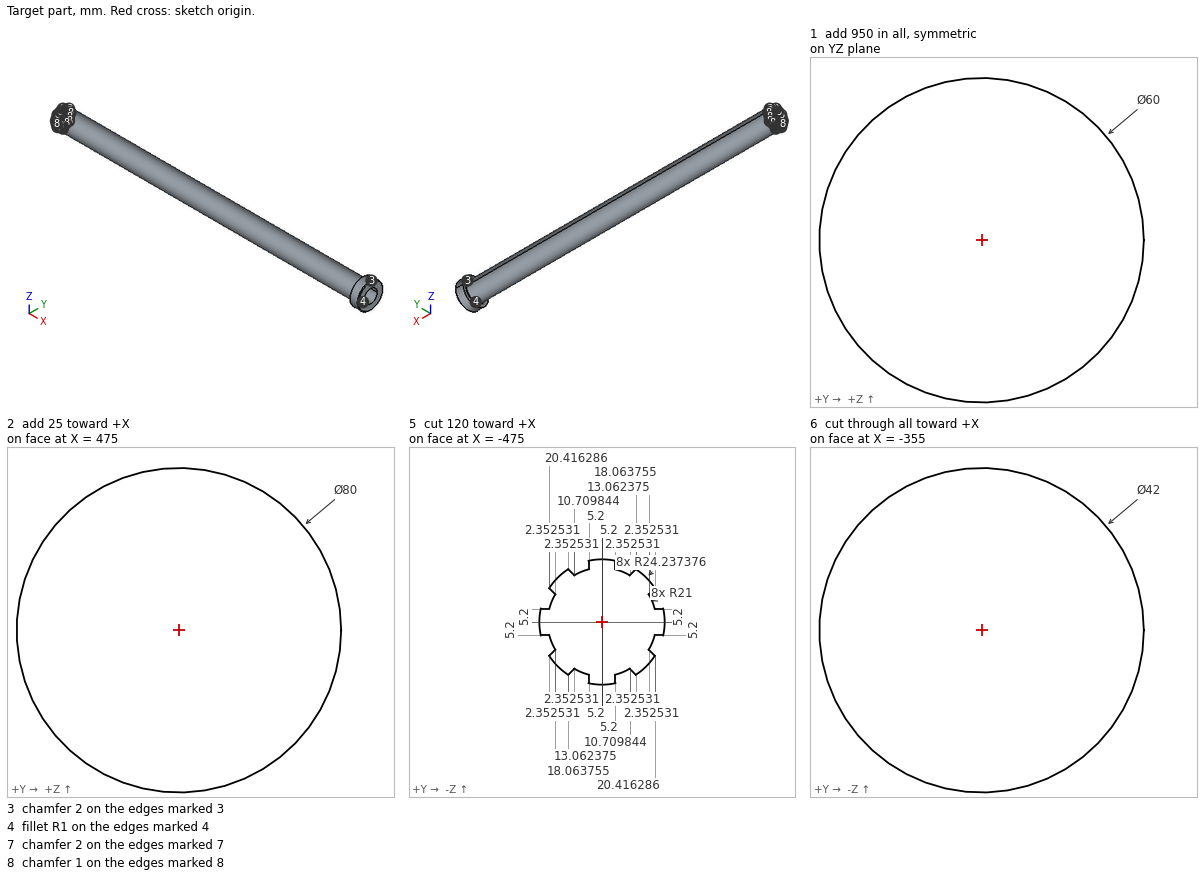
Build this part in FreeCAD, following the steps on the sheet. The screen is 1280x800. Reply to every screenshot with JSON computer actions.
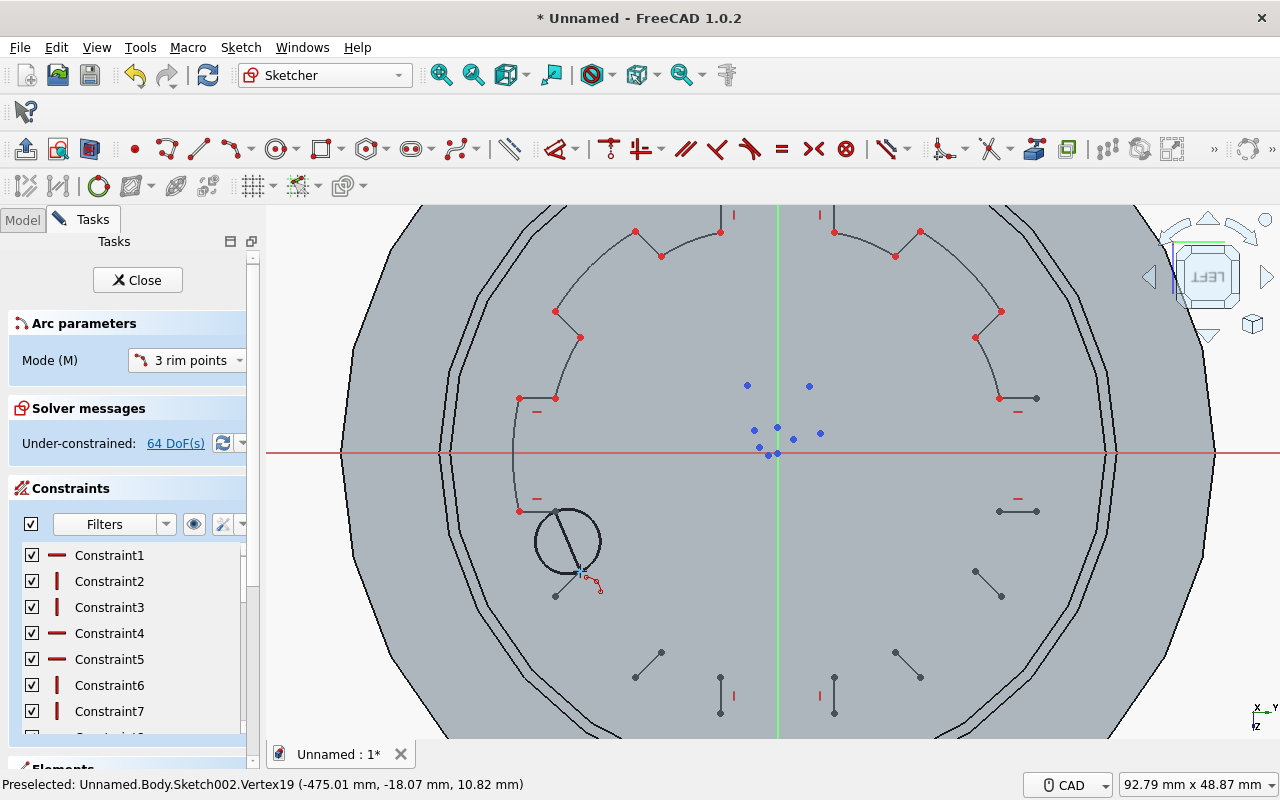
{"action": "scroll", "coordinate": [566, 541], "scroll_direction": "up", "scroll_amount": 10}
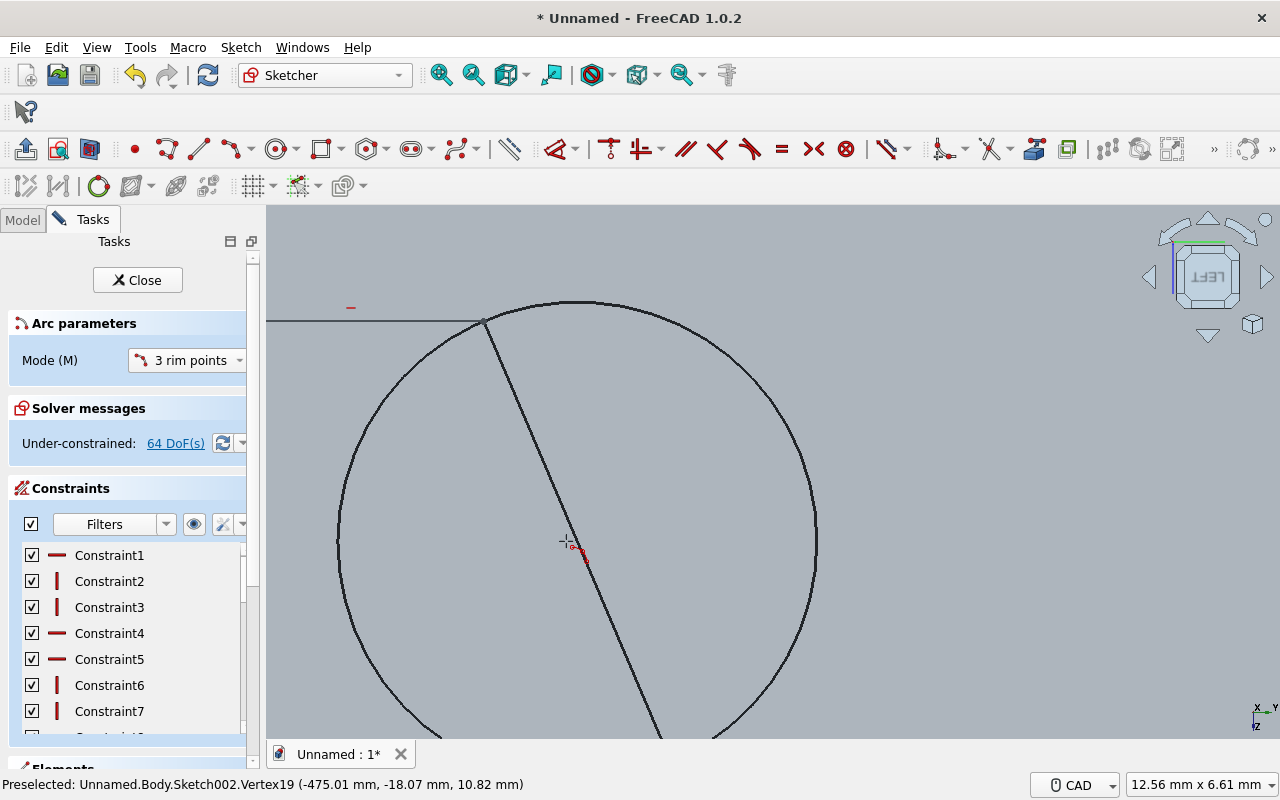
{"action": "left_click", "coordinate": [564, 537]}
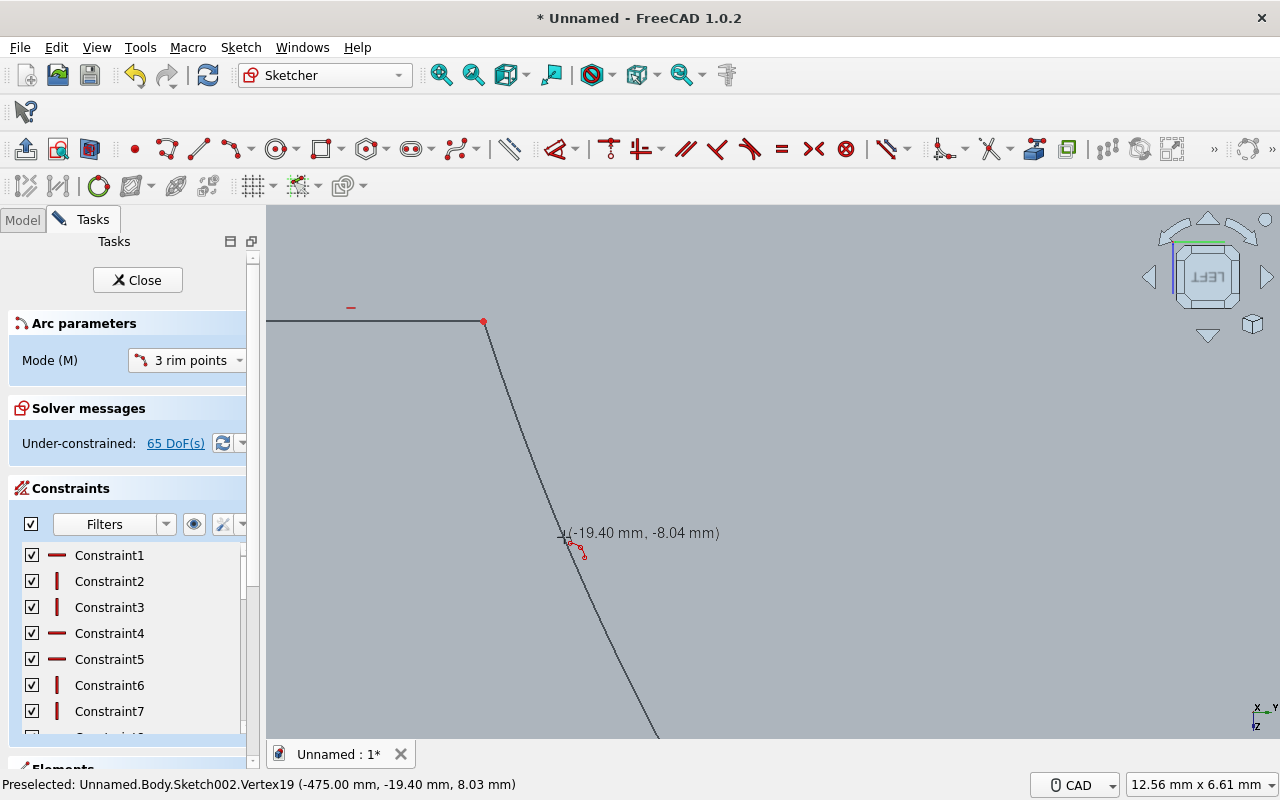
{"action": "scroll", "coordinate": [562, 530], "scroll_direction": "down", "scroll_amount": 12}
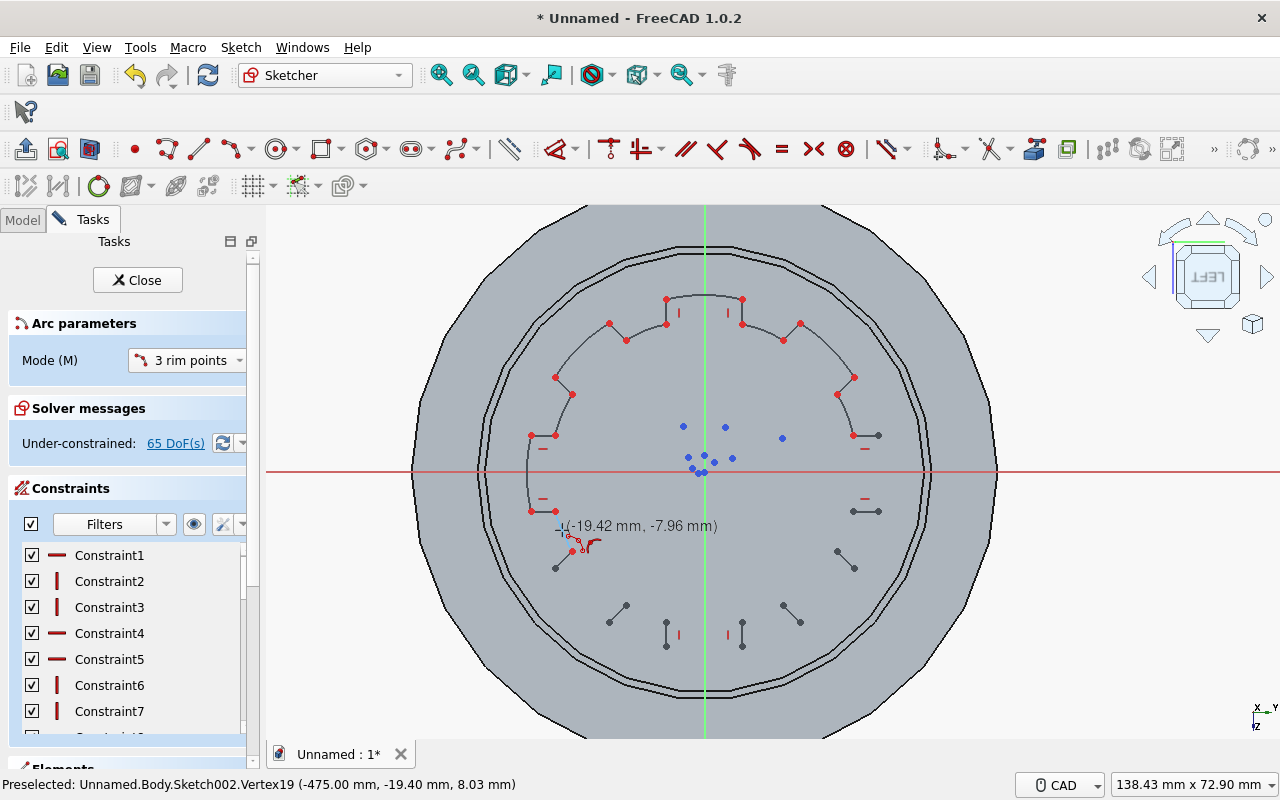
{"action": "scroll", "coordinate": [555, 568], "scroll_direction": "up", "scroll_amount": 2}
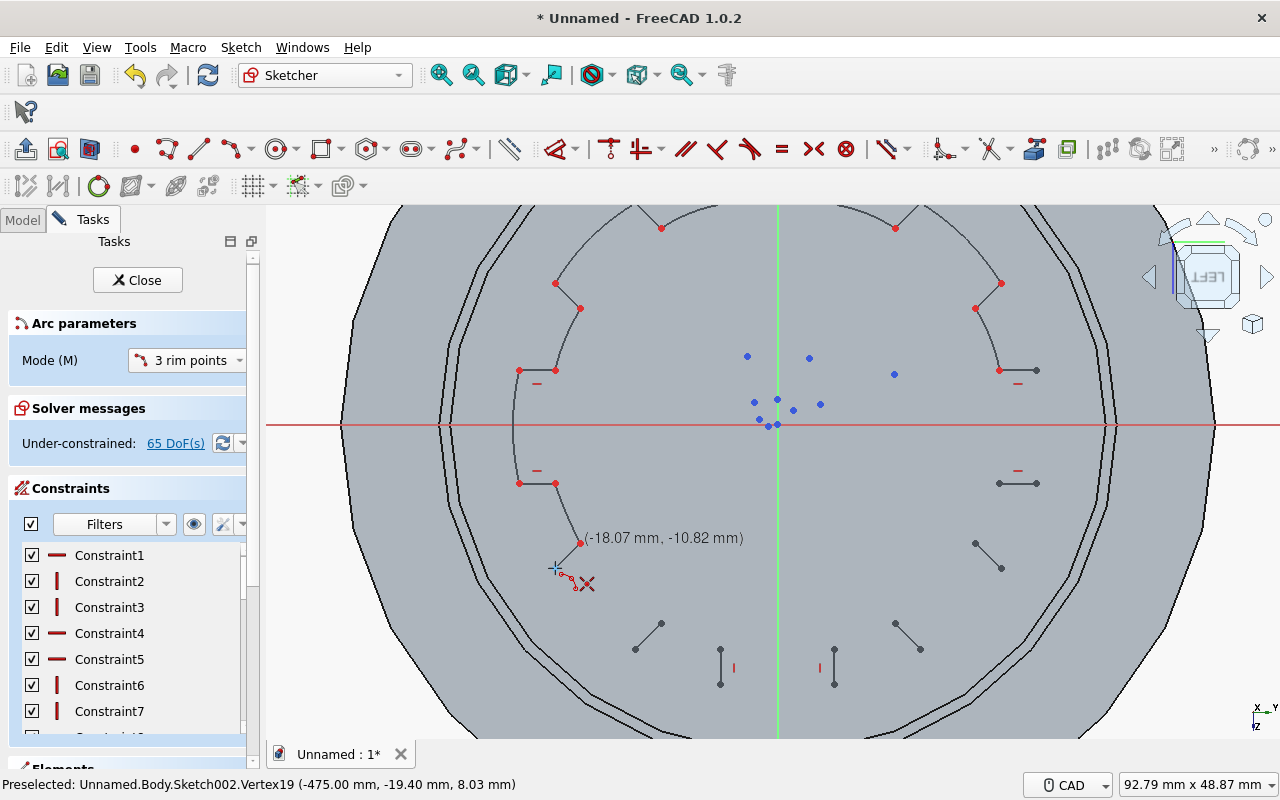
{"action": "left_click", "coordinate": [555, 569]}
{"action": "left_click", "coordinate": [636, 649]}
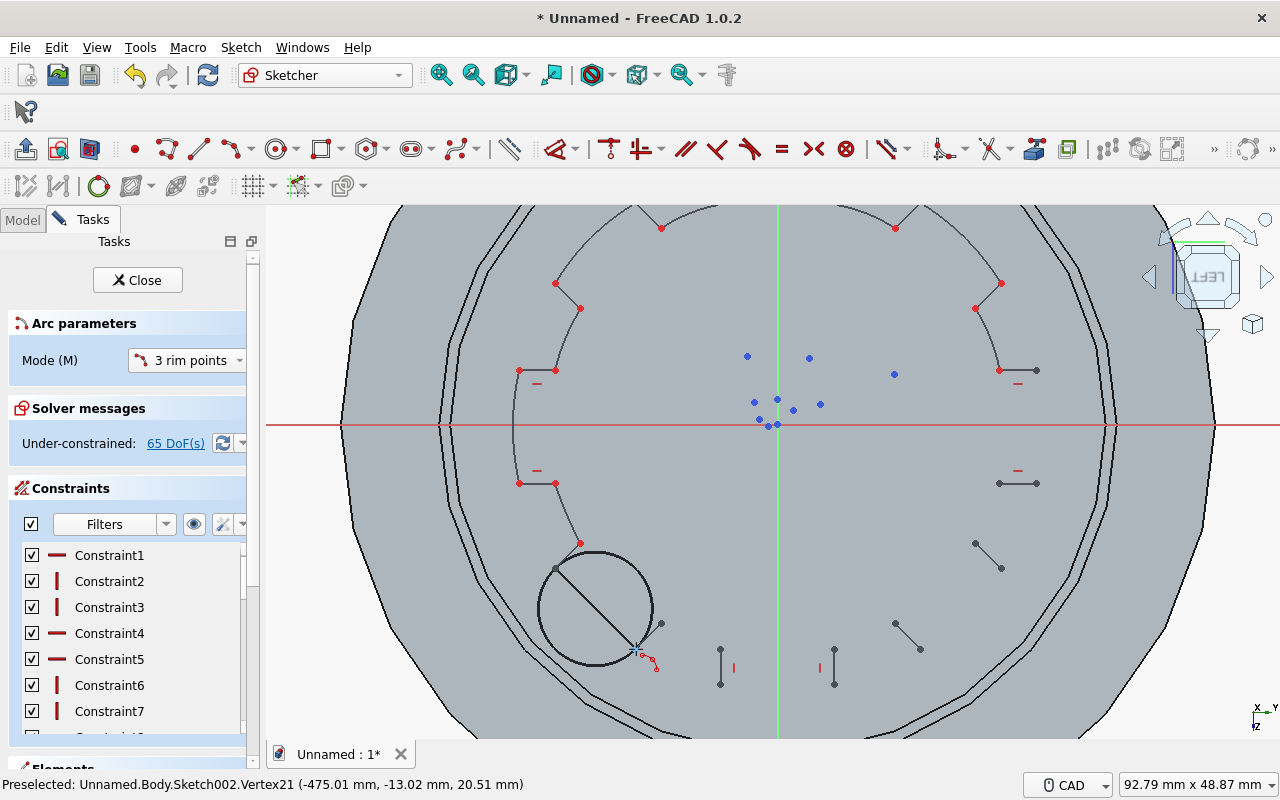
{"action": "scroll", "coordinate": [591, 612], "scroll_direction": "up", "scroll_amount": 5}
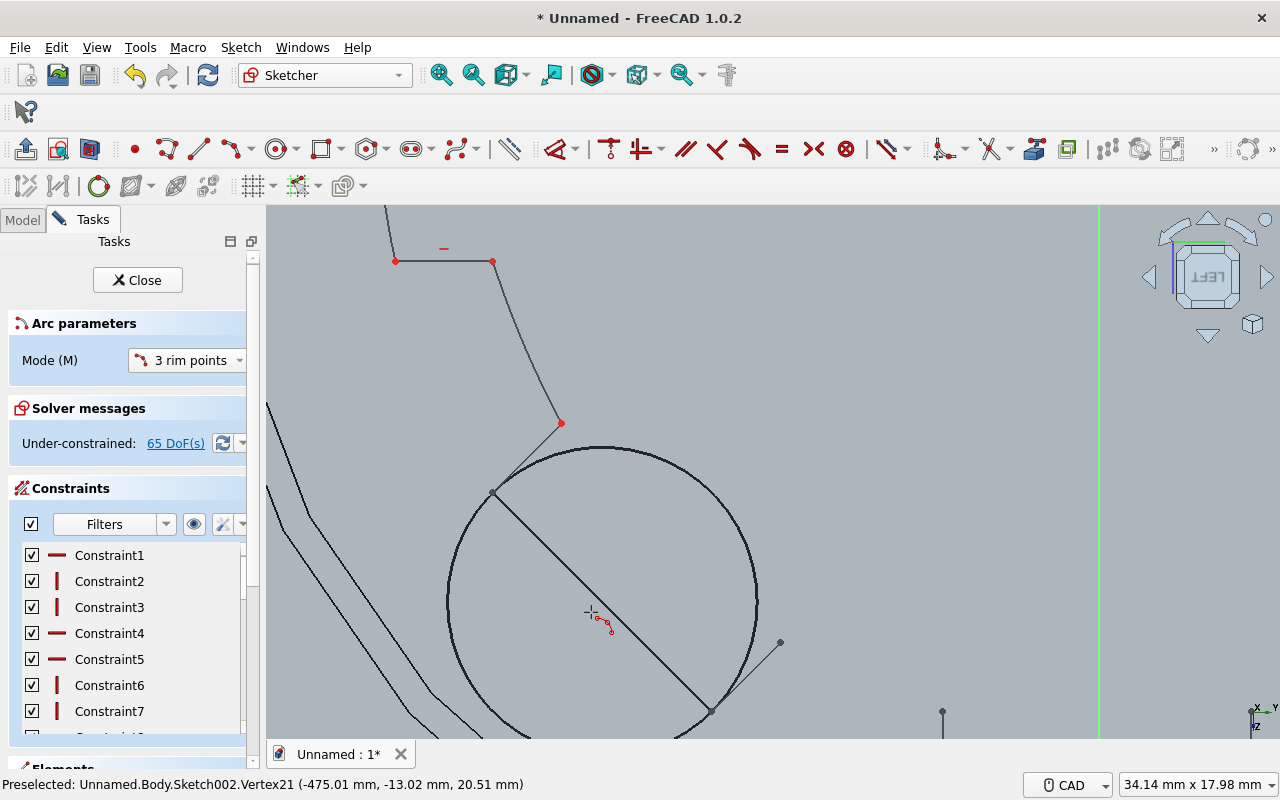
{"action": "left_click", "coordinate": [590, 611]}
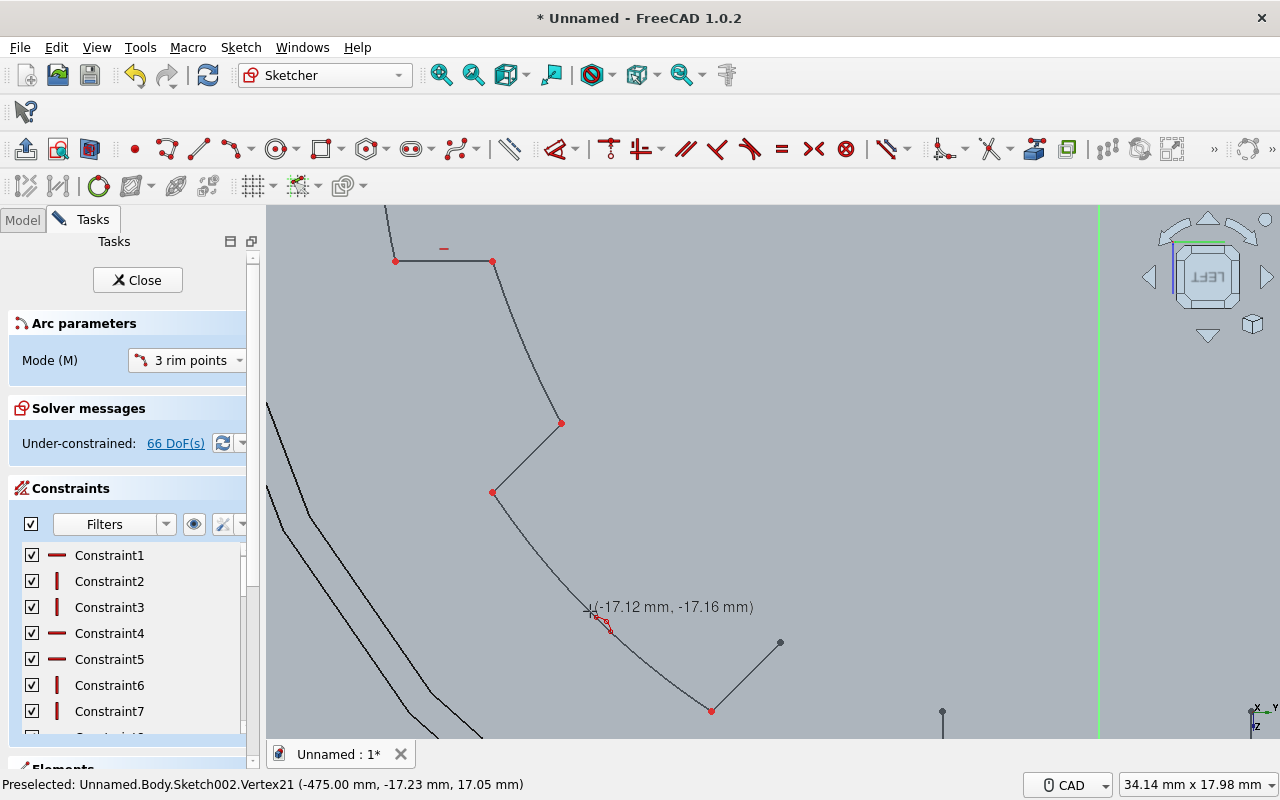
{"action": "scroll", "coordinate": [575, 593], "scroll_direction": "down", "scroll_amount": 7}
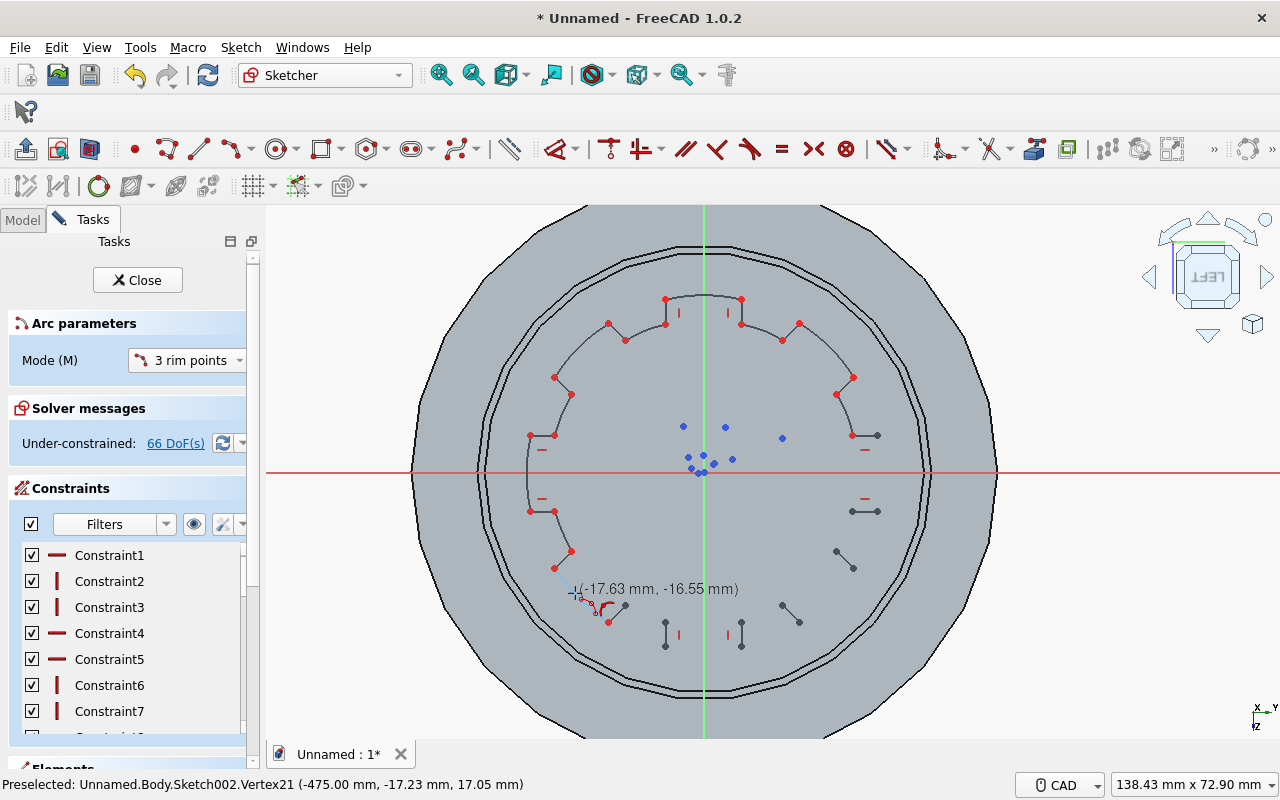
{"action": "scroll", "coordinate": [626, 605], "scroll_direction": "up", "scroll_amount": 2}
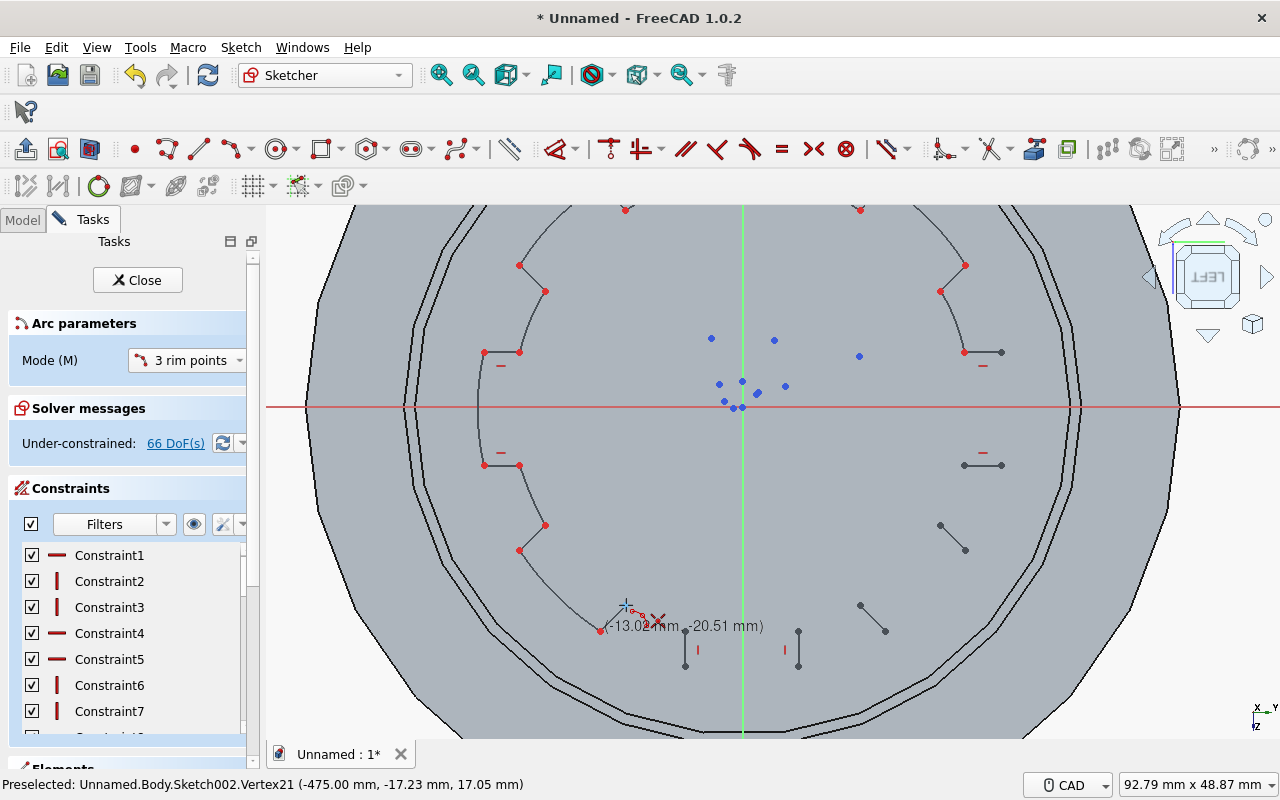
{"action": "left_click", "coordinate": [626, 606]}
{"action": "left_click", "coordinate": [685, 631]}